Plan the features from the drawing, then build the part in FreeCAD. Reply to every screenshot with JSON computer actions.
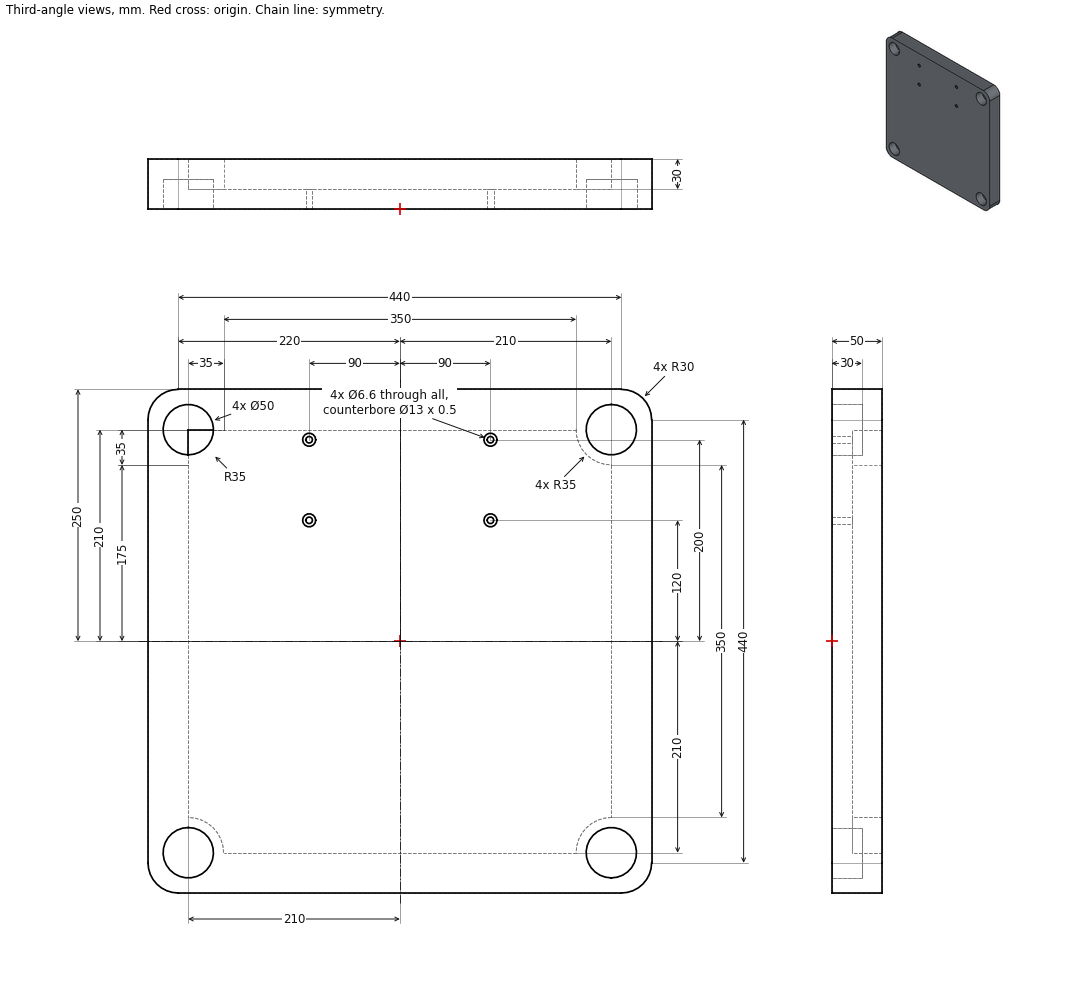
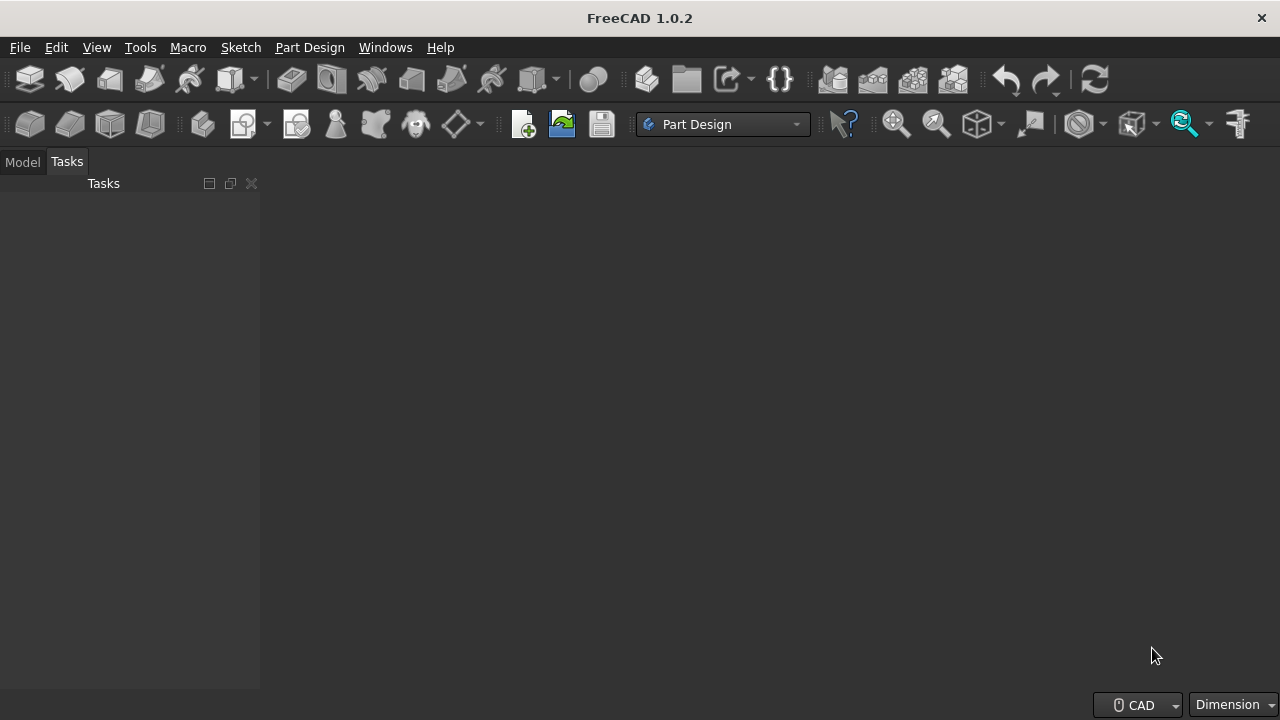
{"action": "left_click", "coordinate": [522, 124]}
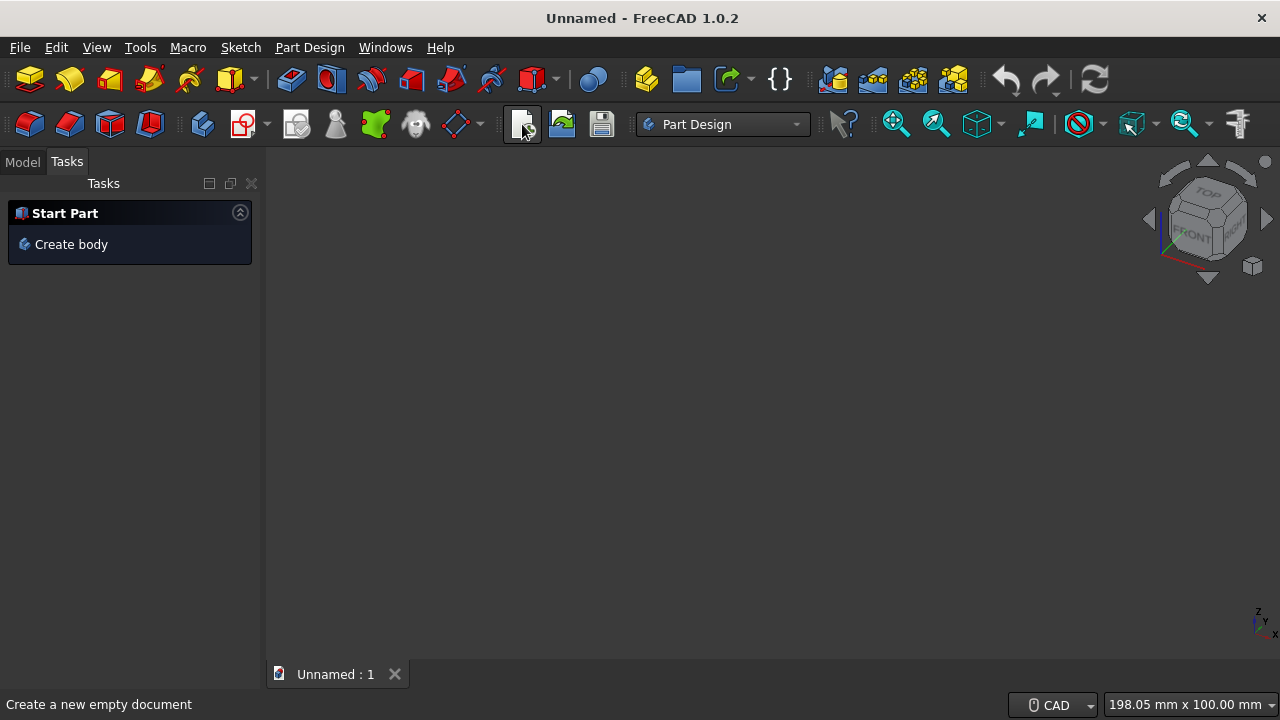
{"action": "left_click", "coordinate": [244, 124]}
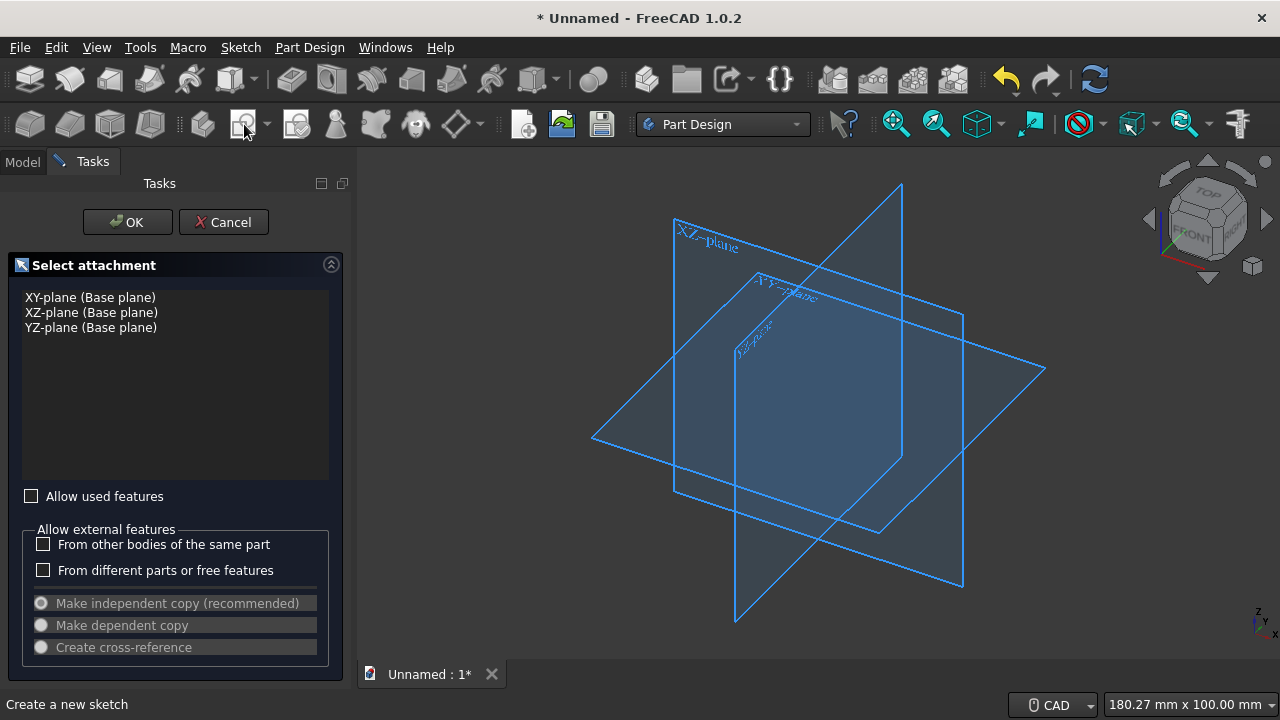
{"action": "left_click", "coordinate": [82, 312]}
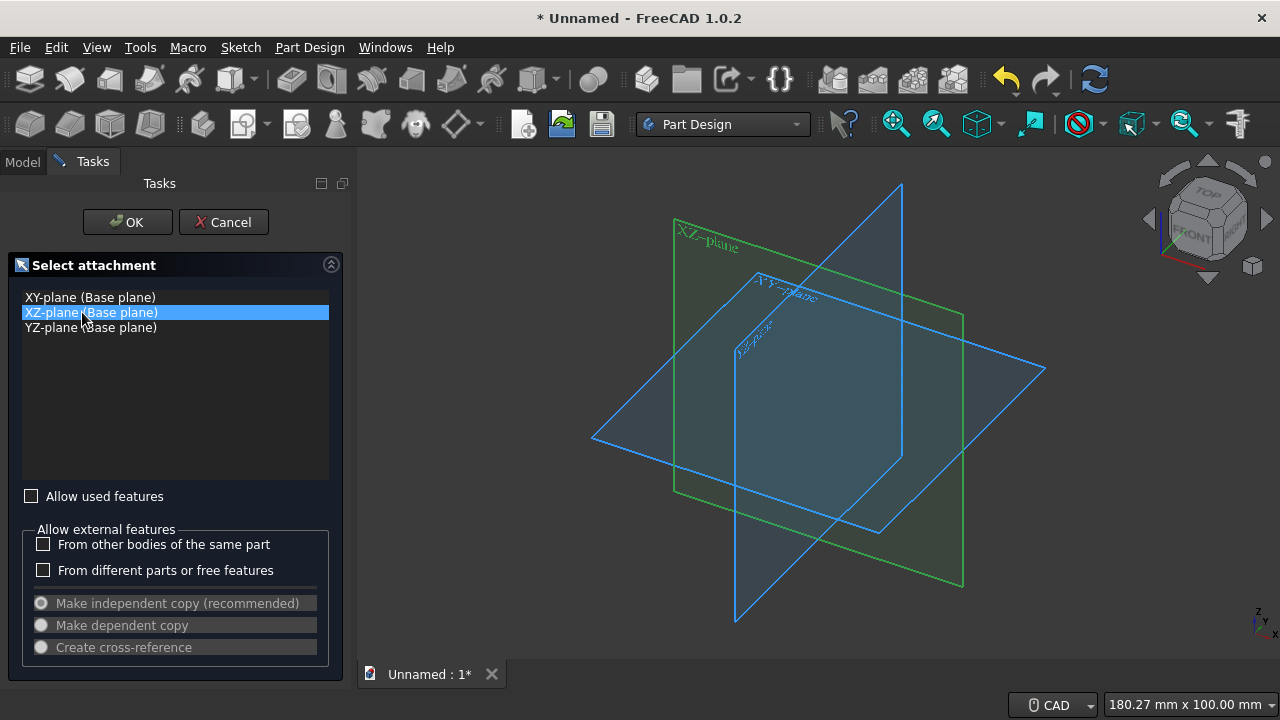
{"action": "left_click", "coordinate": [128, 222]}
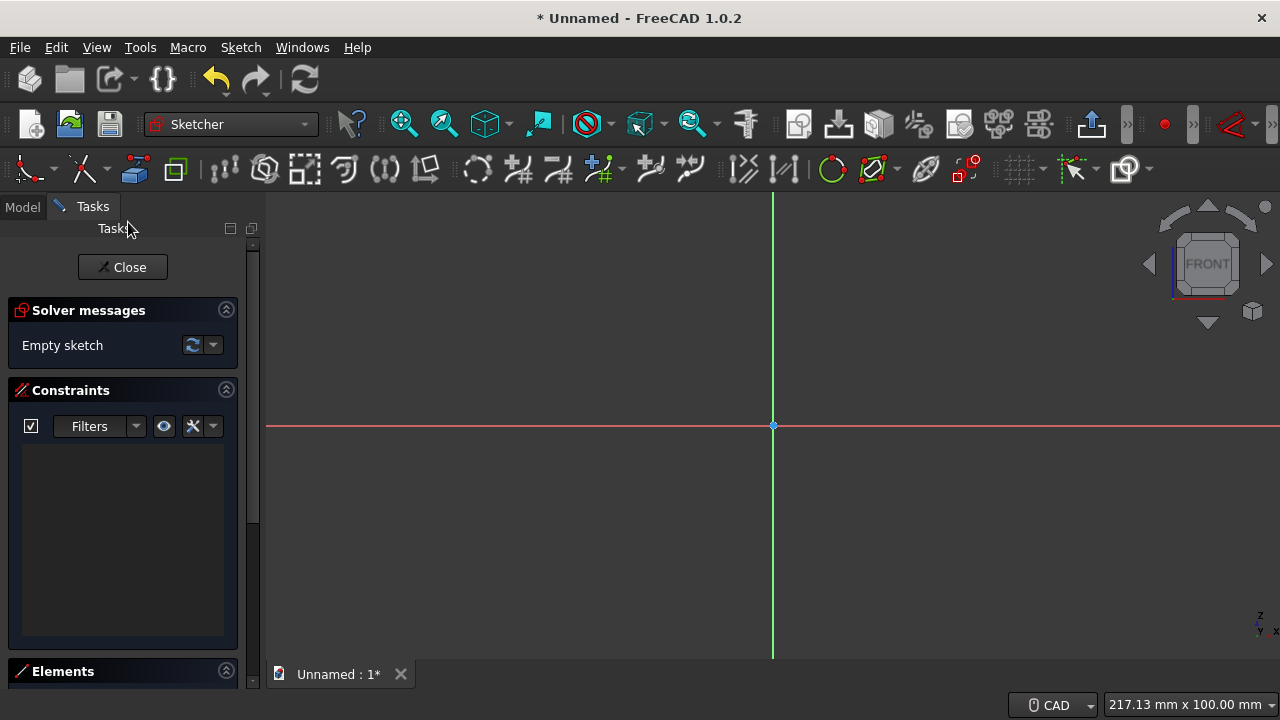
{"action": "scroll", "coordinate": [694, 426], "scroll_direction": "down", "scroll_amount": 10}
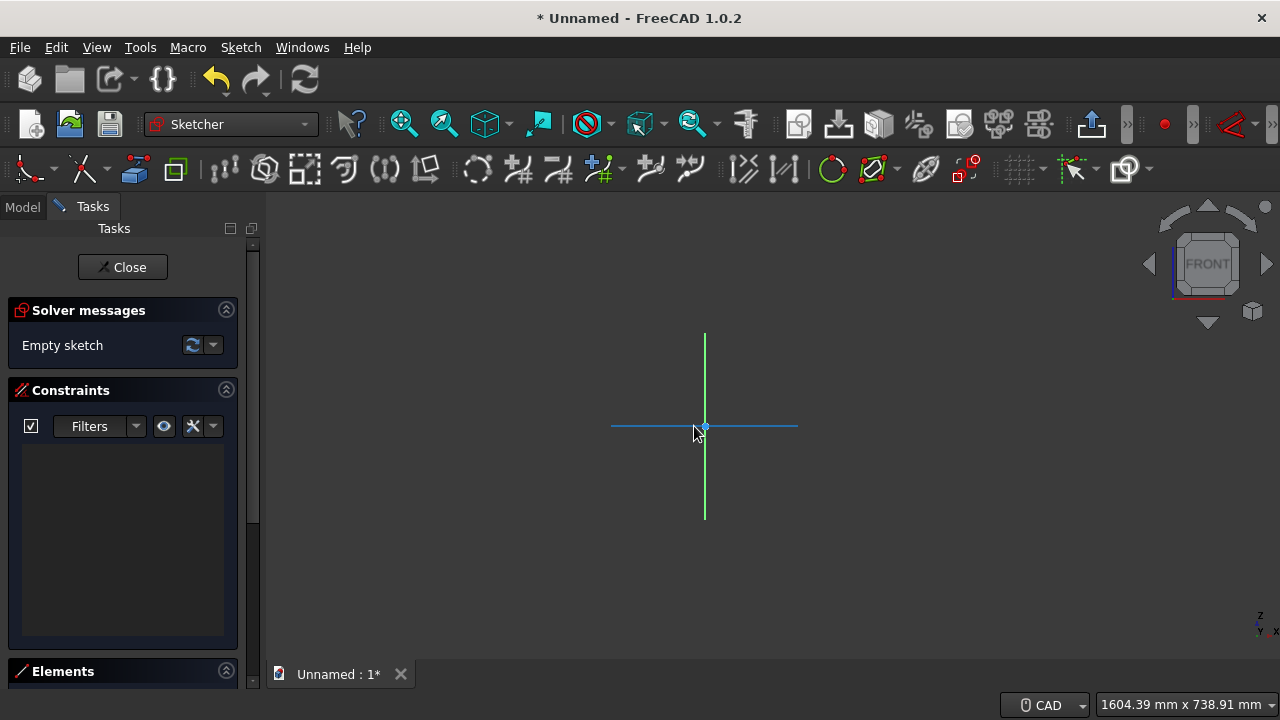
{"action": "key", "text": "g l"}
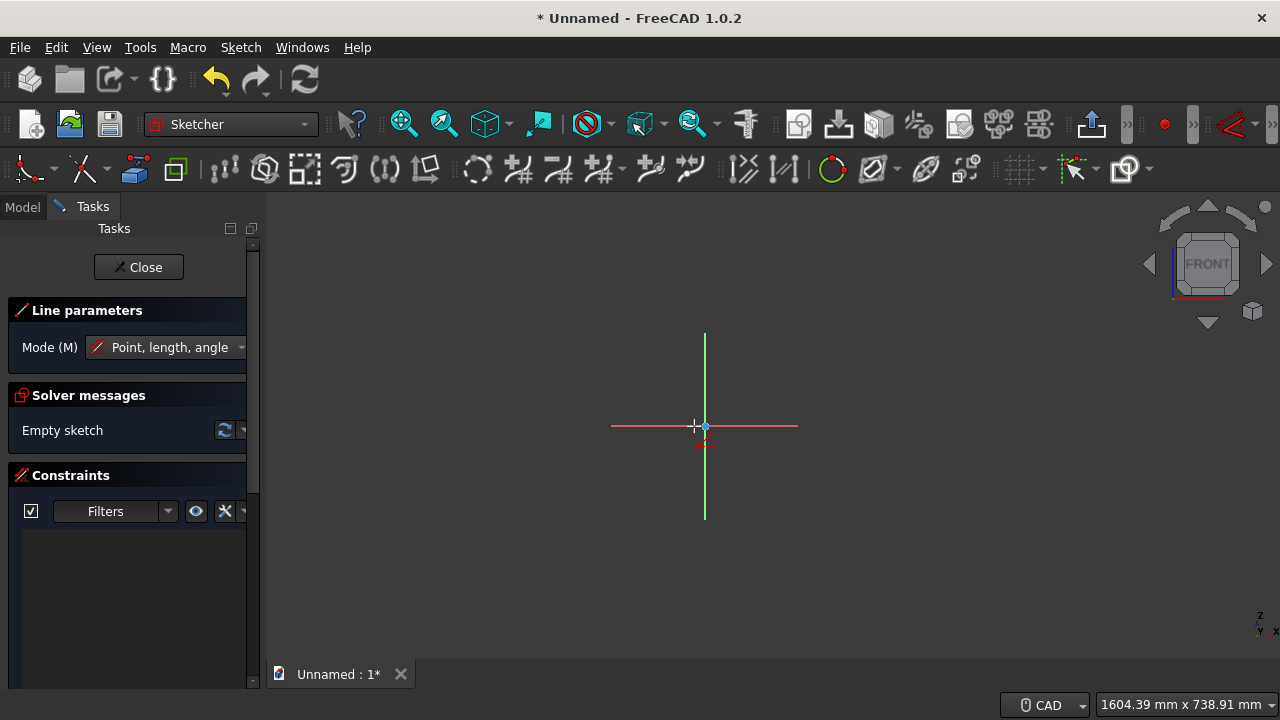
{"action": "left_click", "coordinate": [566, 268]}
{"action": "left_click", "coordinate": [844, 268]}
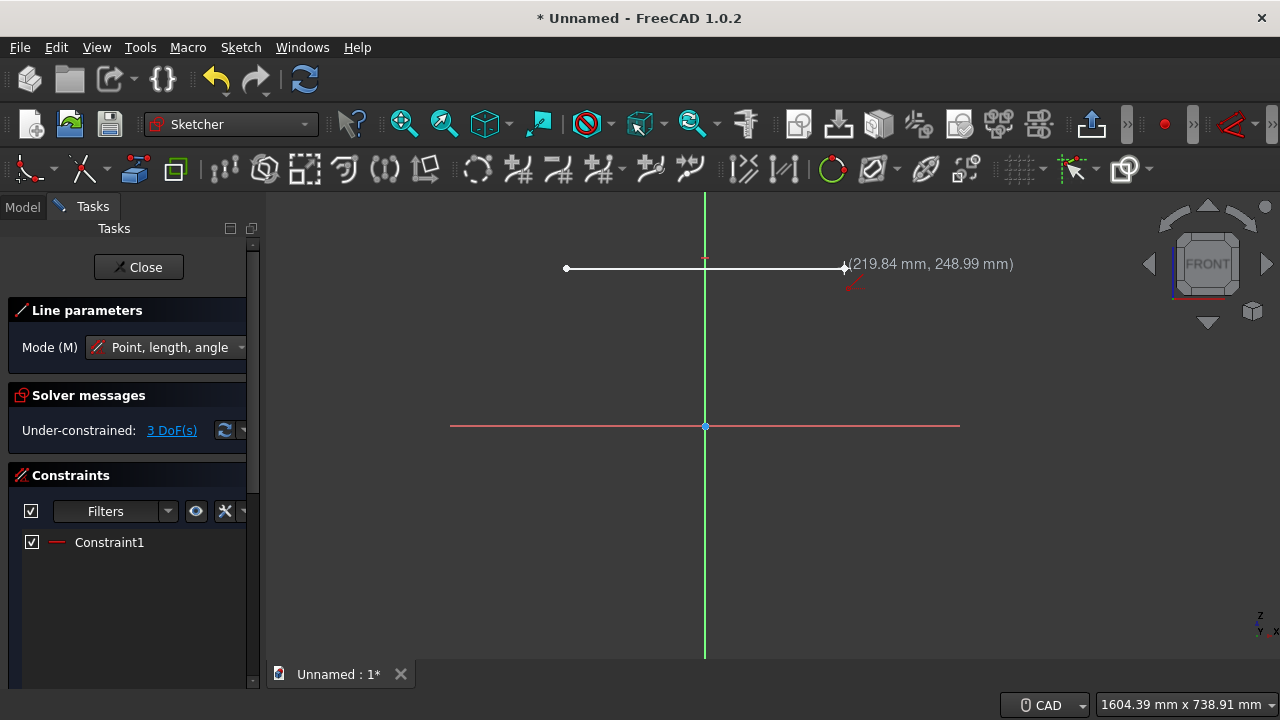
{"action": "left_click", "coordinate": [863, 287]}
{"action": "left_click", "coordinate": [863, 565]}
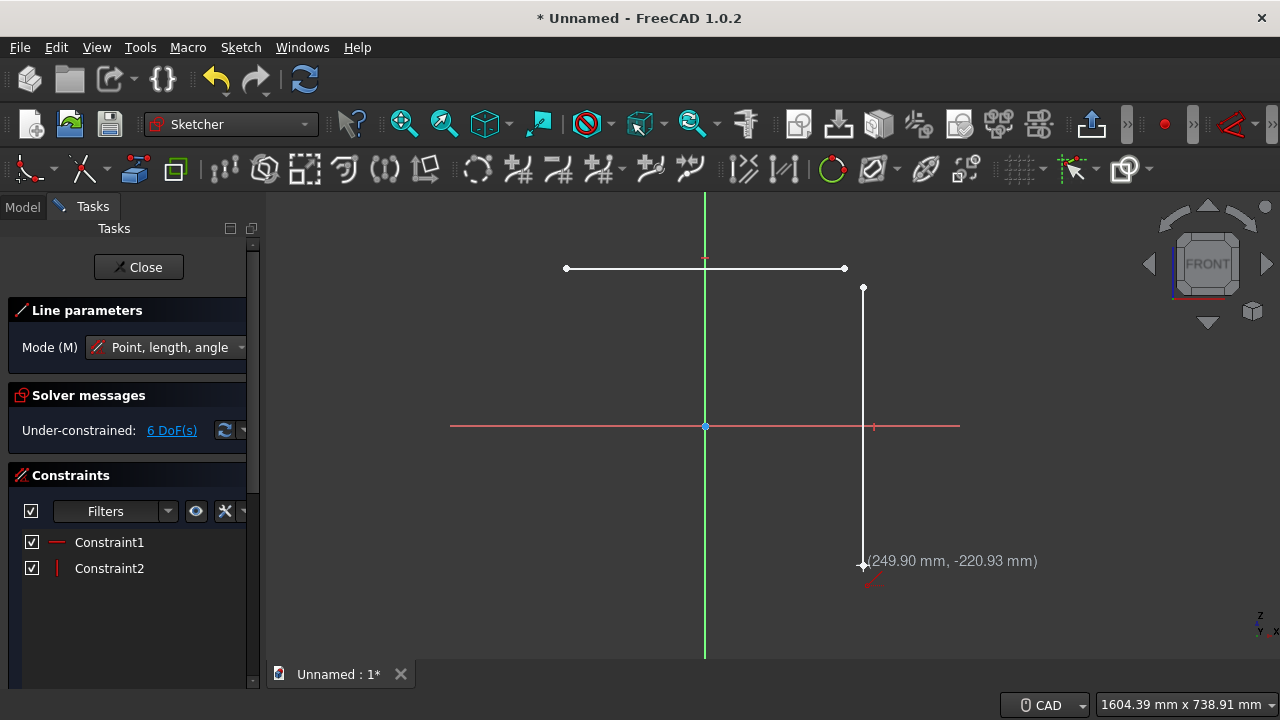
{"action": "left_click", "coordinate": [844, 584]}
{"action": "left_click", "coordinate": [566, 584]}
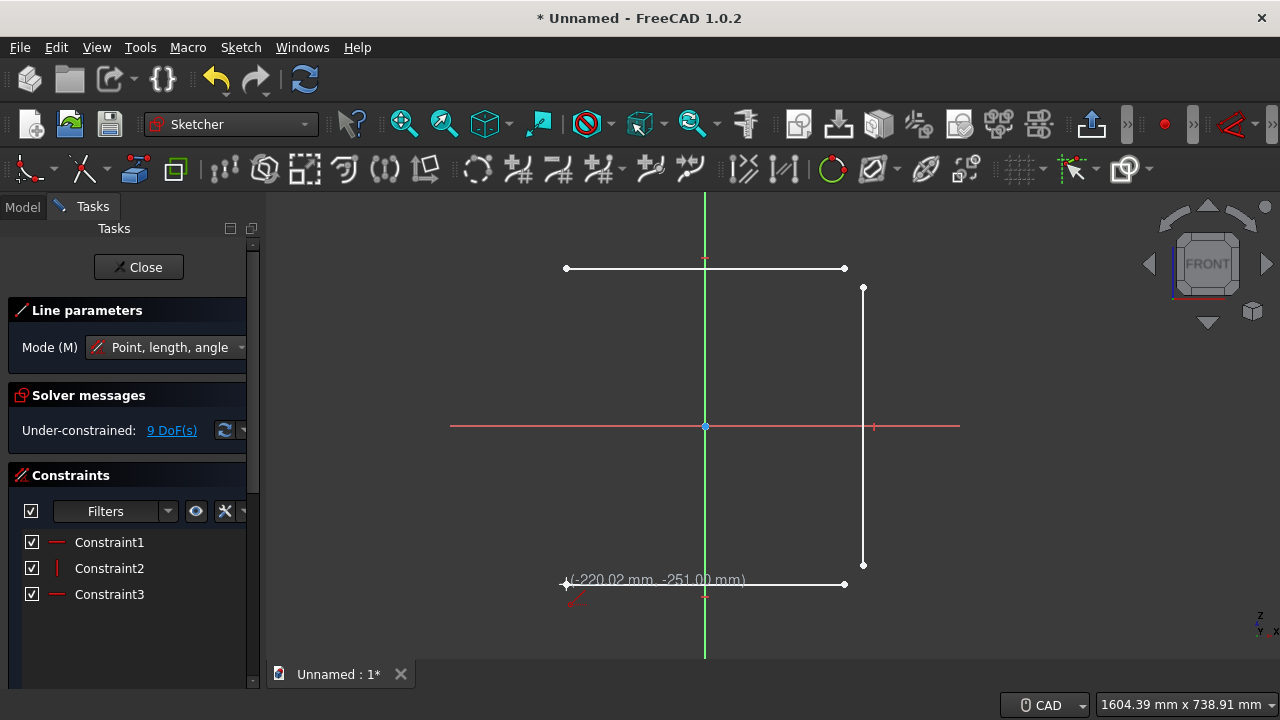
{"action": "left_click", "coordinate": [547, 565]}
{"action": "left_click", "coordinate": [547, 287]}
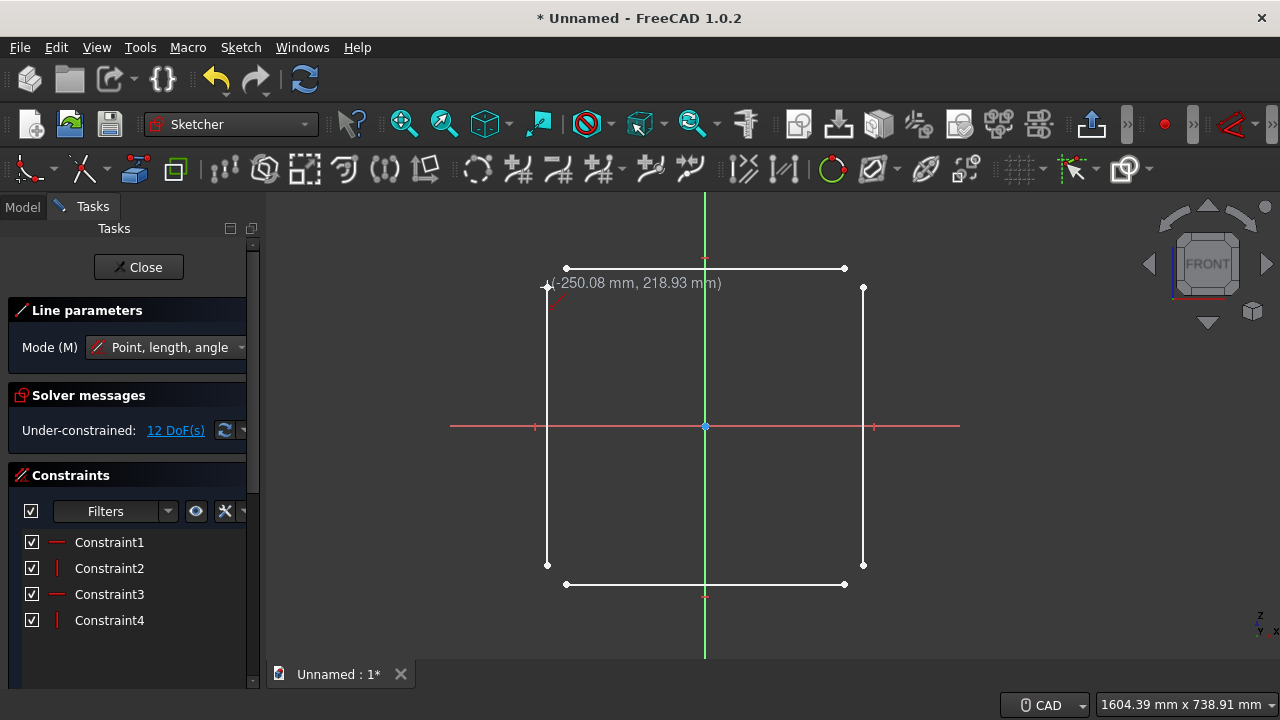
{"action": "key", "text": "g 3 a"}